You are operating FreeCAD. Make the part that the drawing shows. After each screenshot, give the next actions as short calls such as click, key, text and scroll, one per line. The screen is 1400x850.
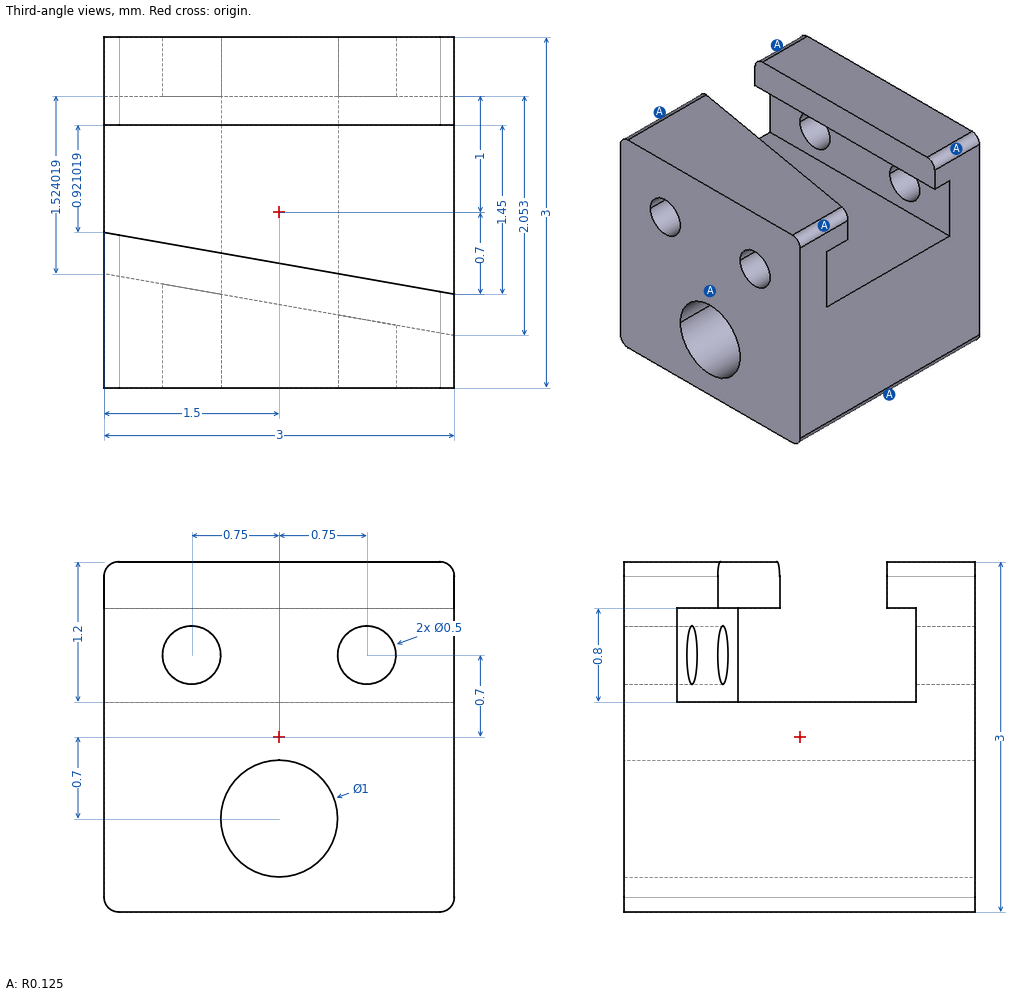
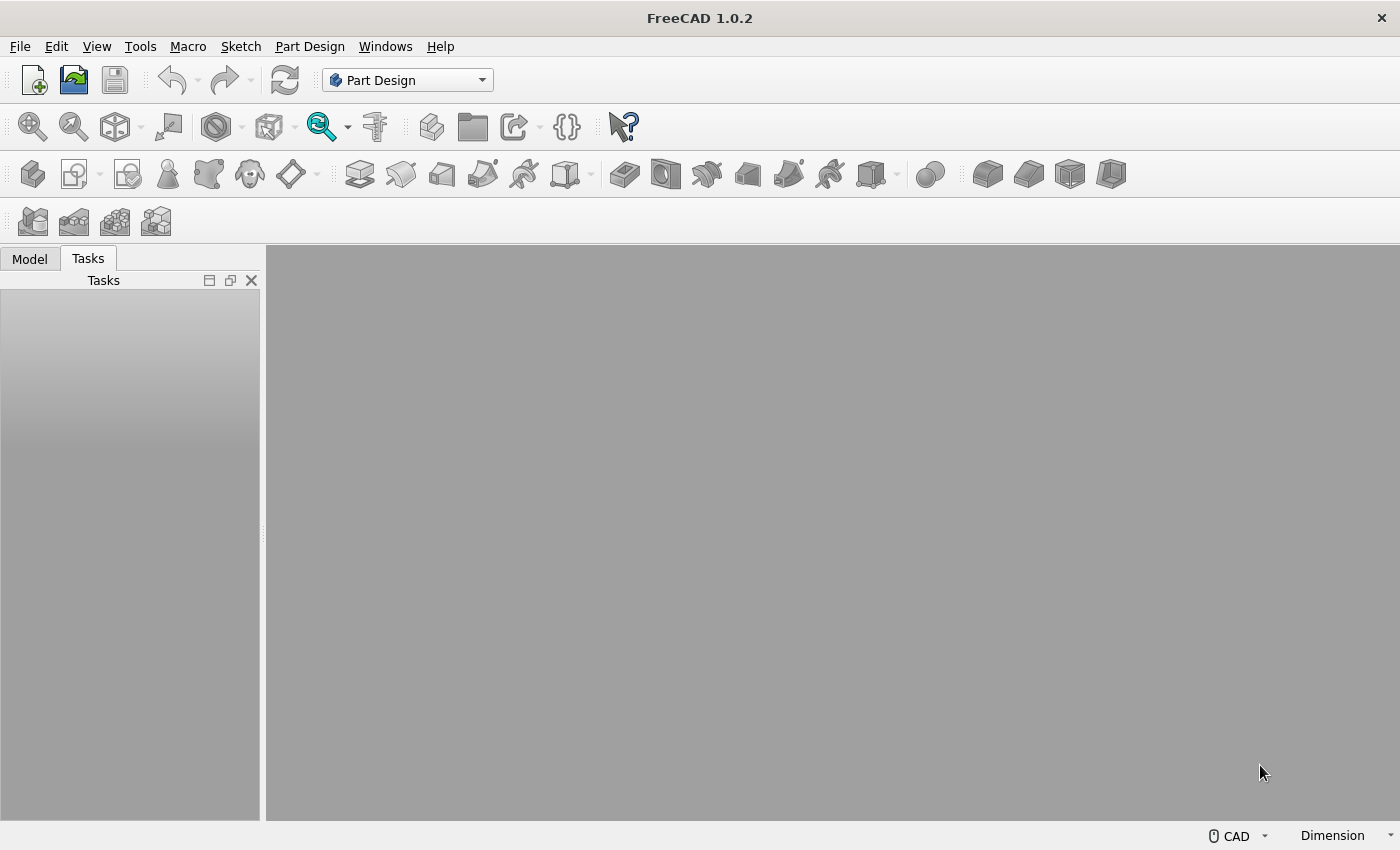
key(ctrl+n)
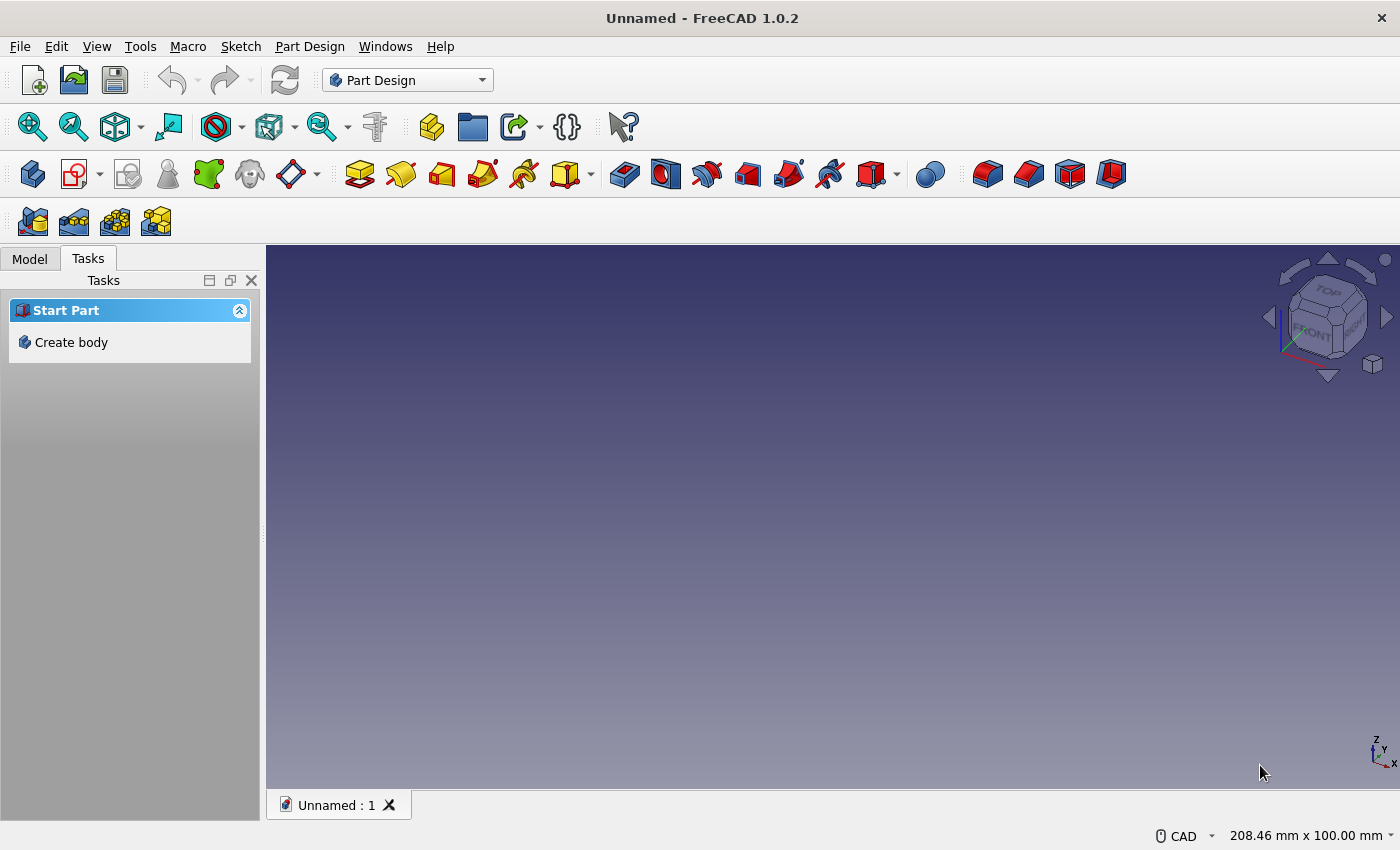
click(74, 174)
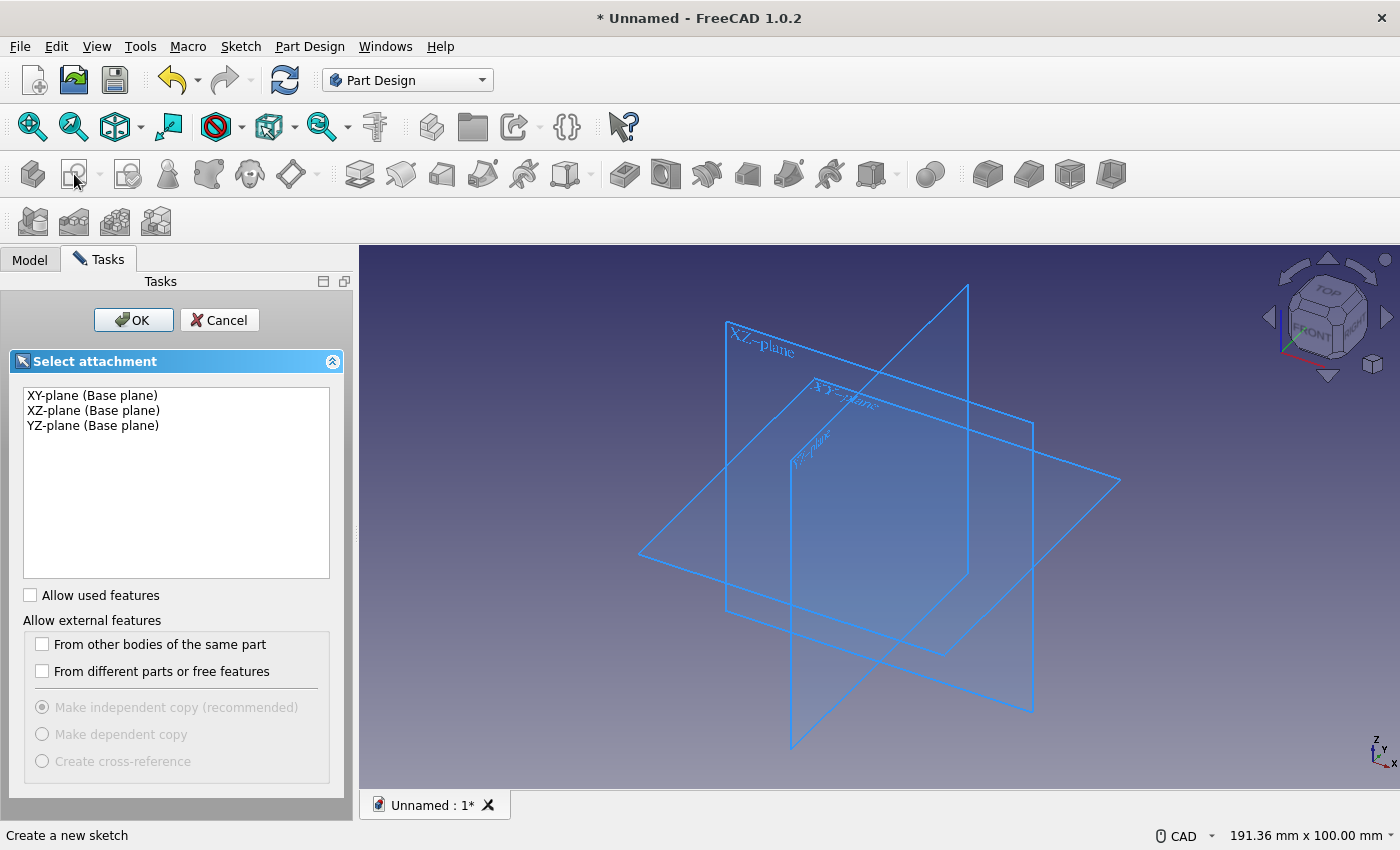
click(84, 396)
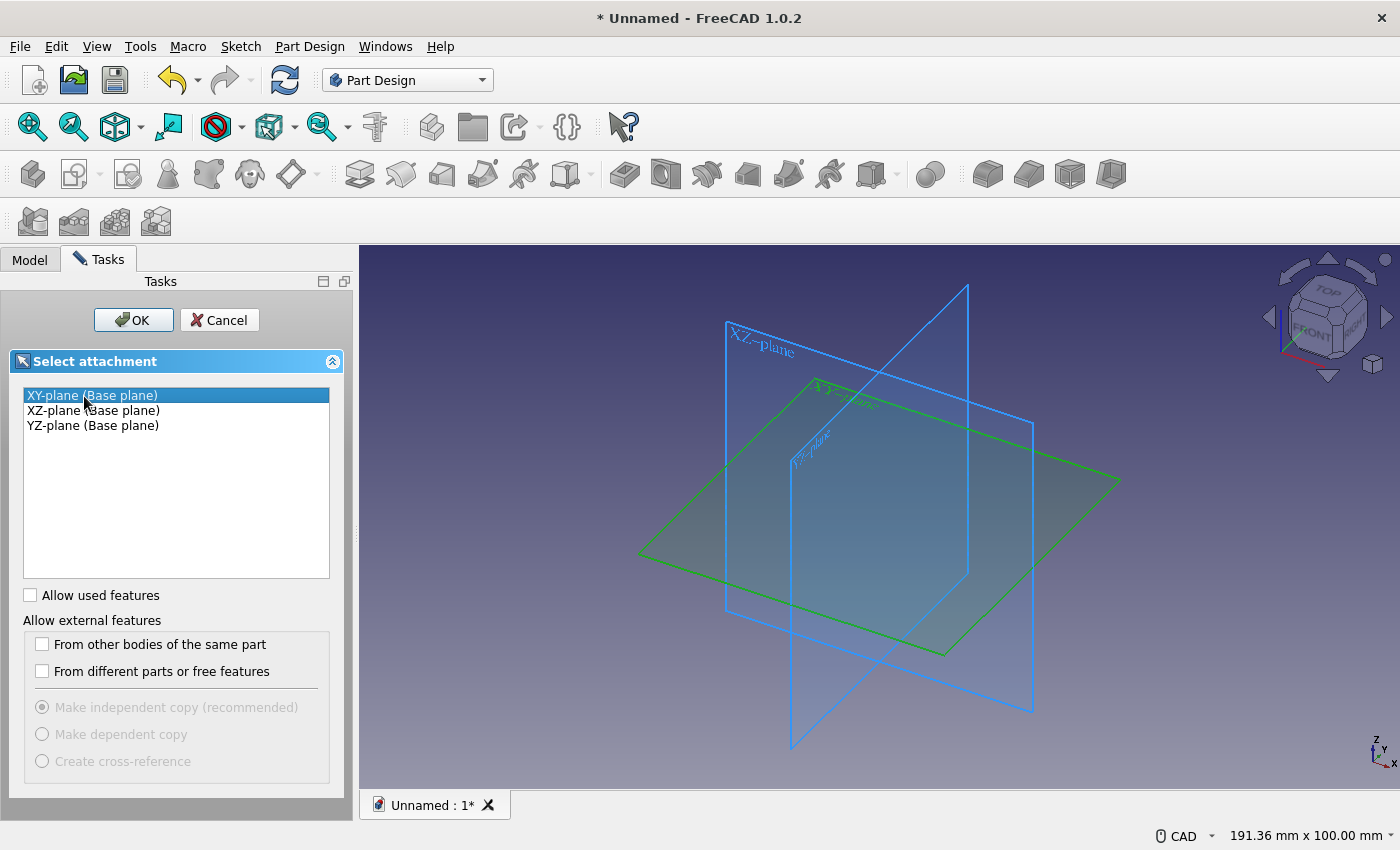
click(134, 320)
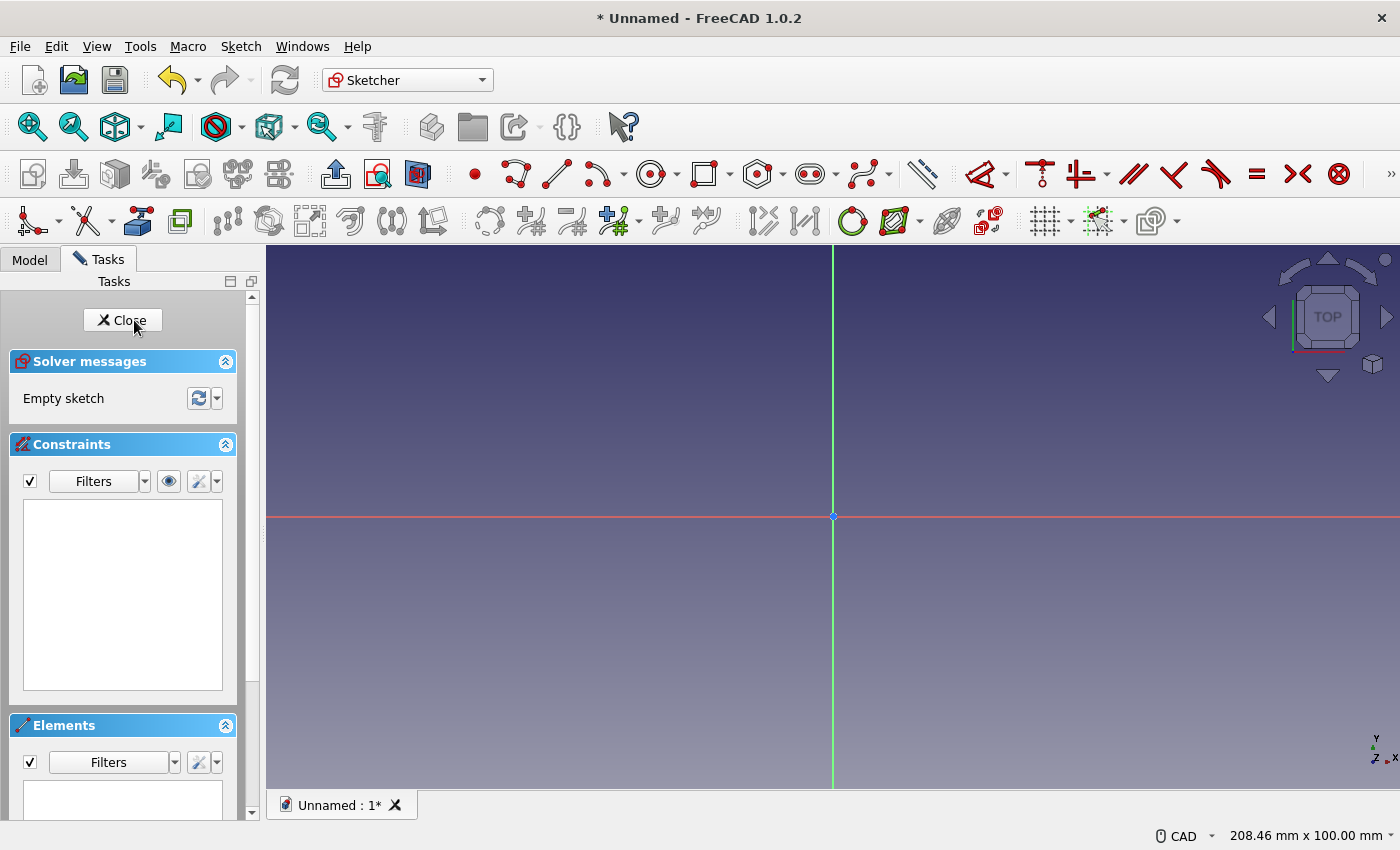
scroll(837, 517, up, 15)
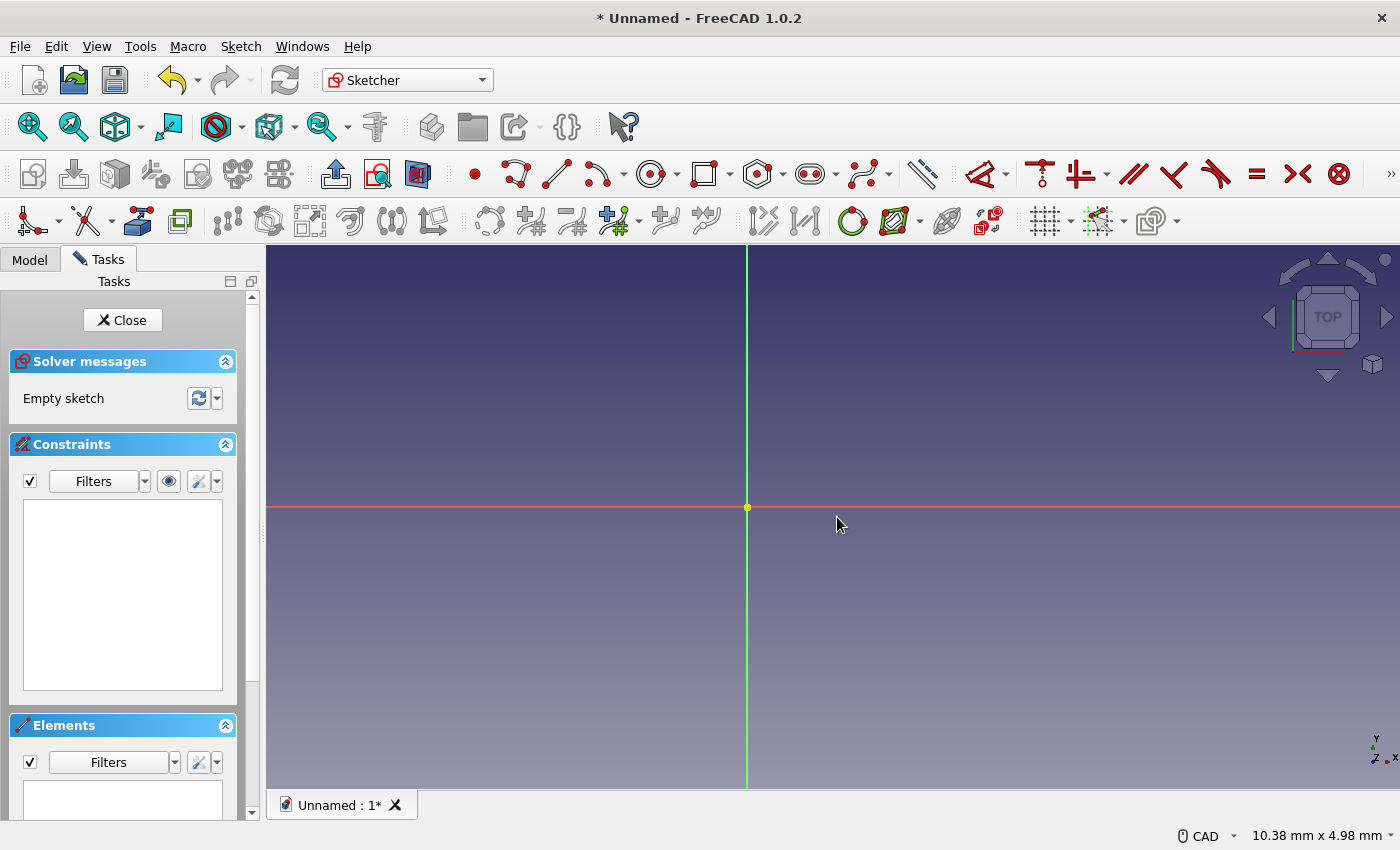
key(g)
key(v)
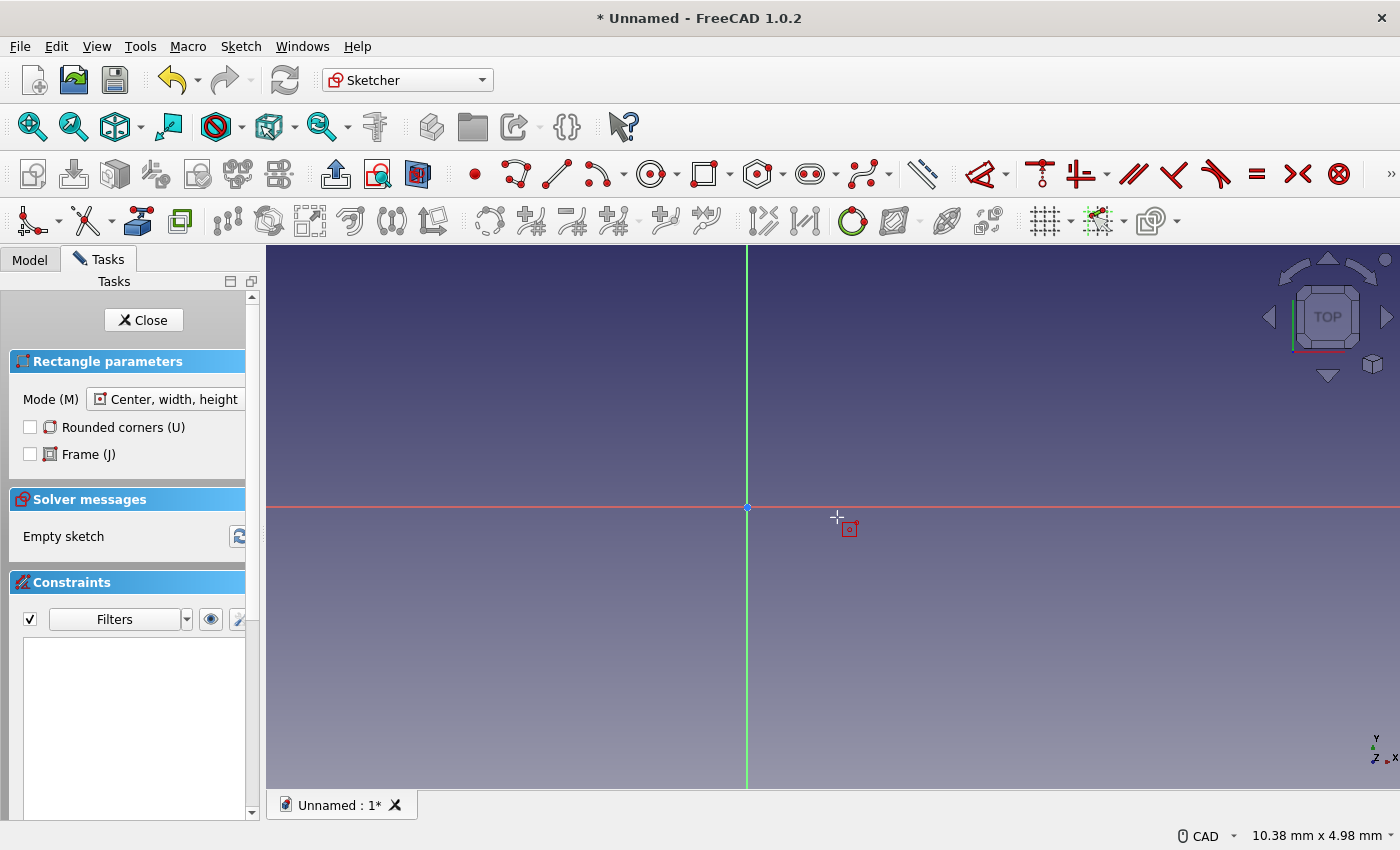
click(747, 507)
click(911, 344)
key(Escape)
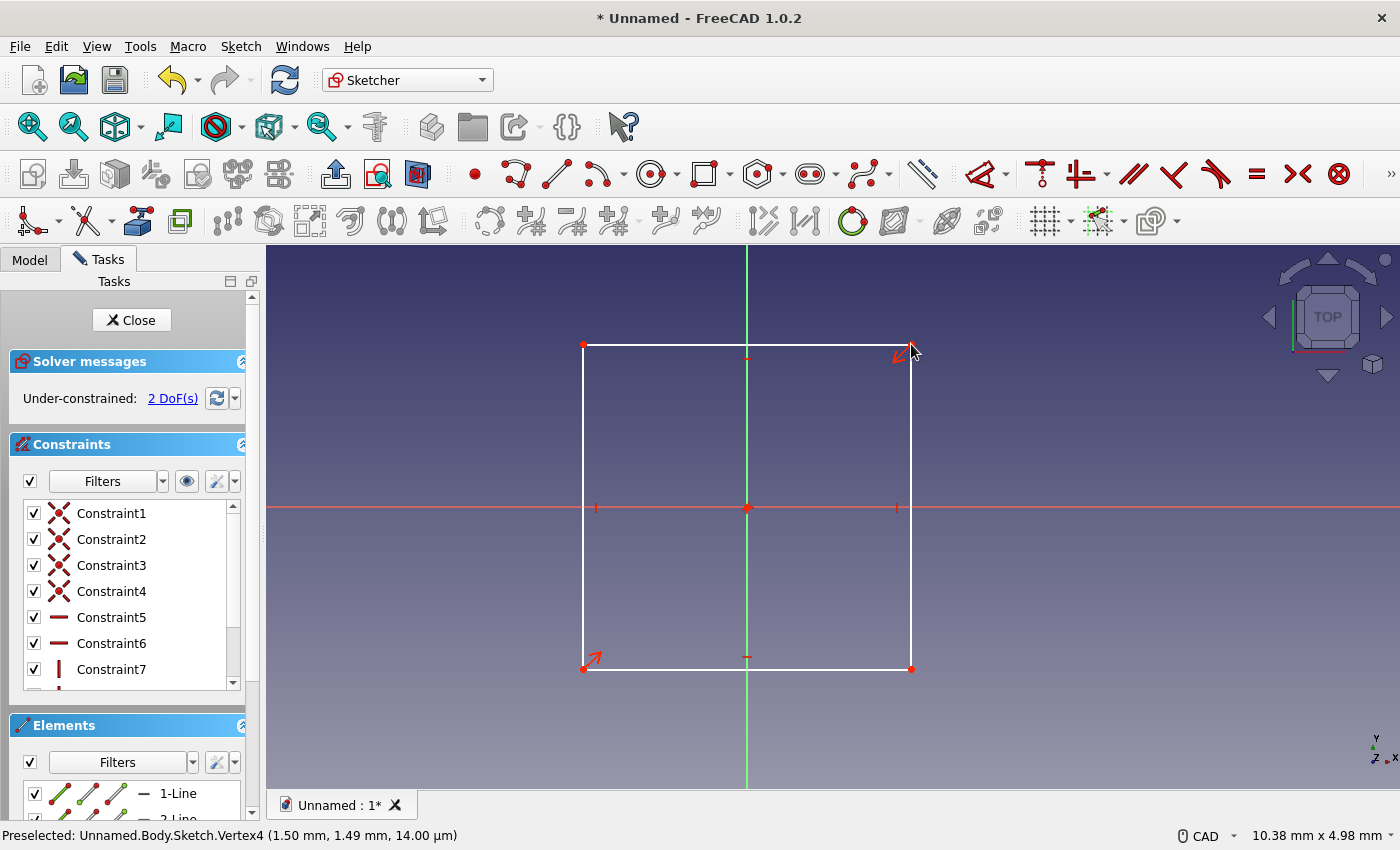
click(980, 174)